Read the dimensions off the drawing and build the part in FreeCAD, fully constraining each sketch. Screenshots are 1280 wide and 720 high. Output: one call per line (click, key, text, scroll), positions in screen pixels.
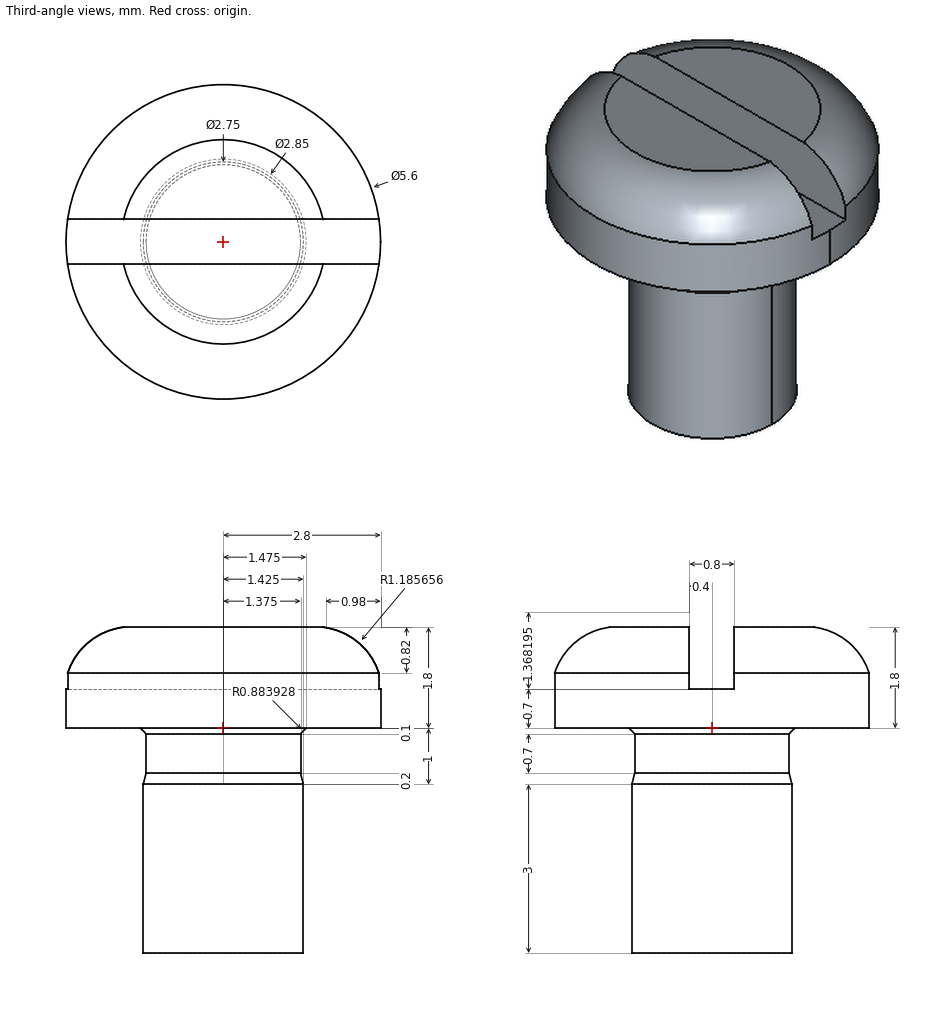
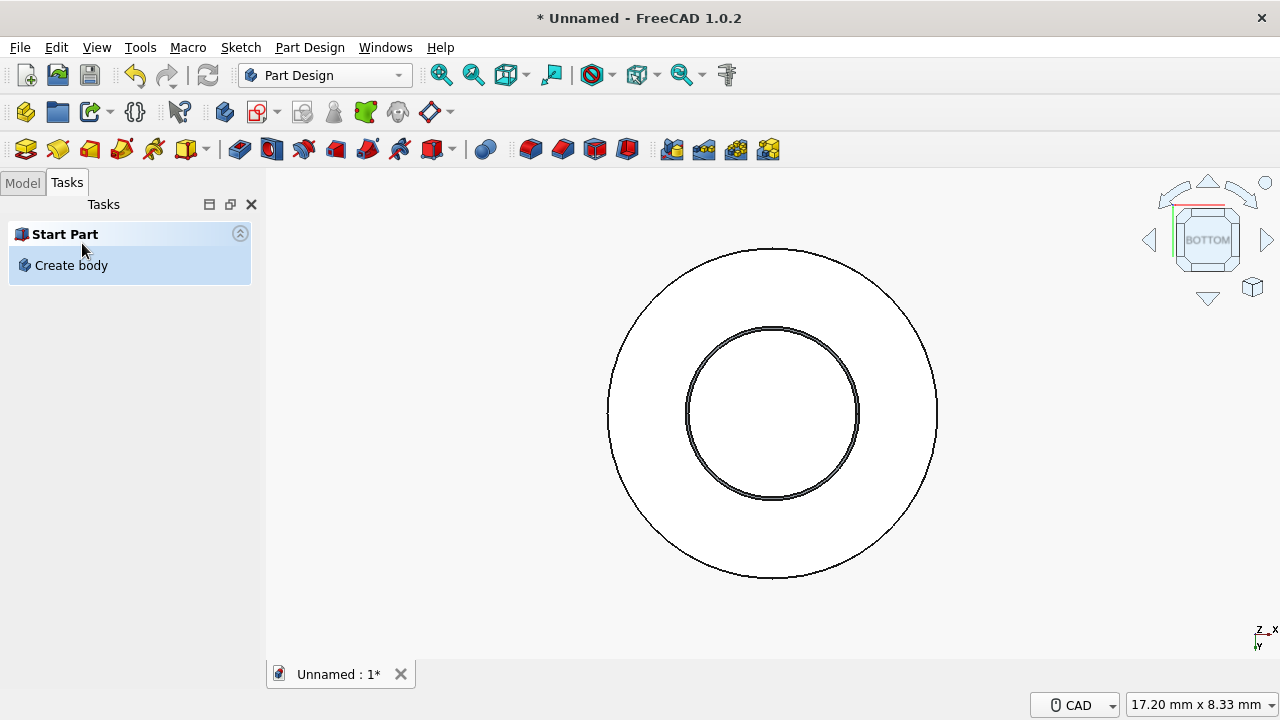
click(23, 182)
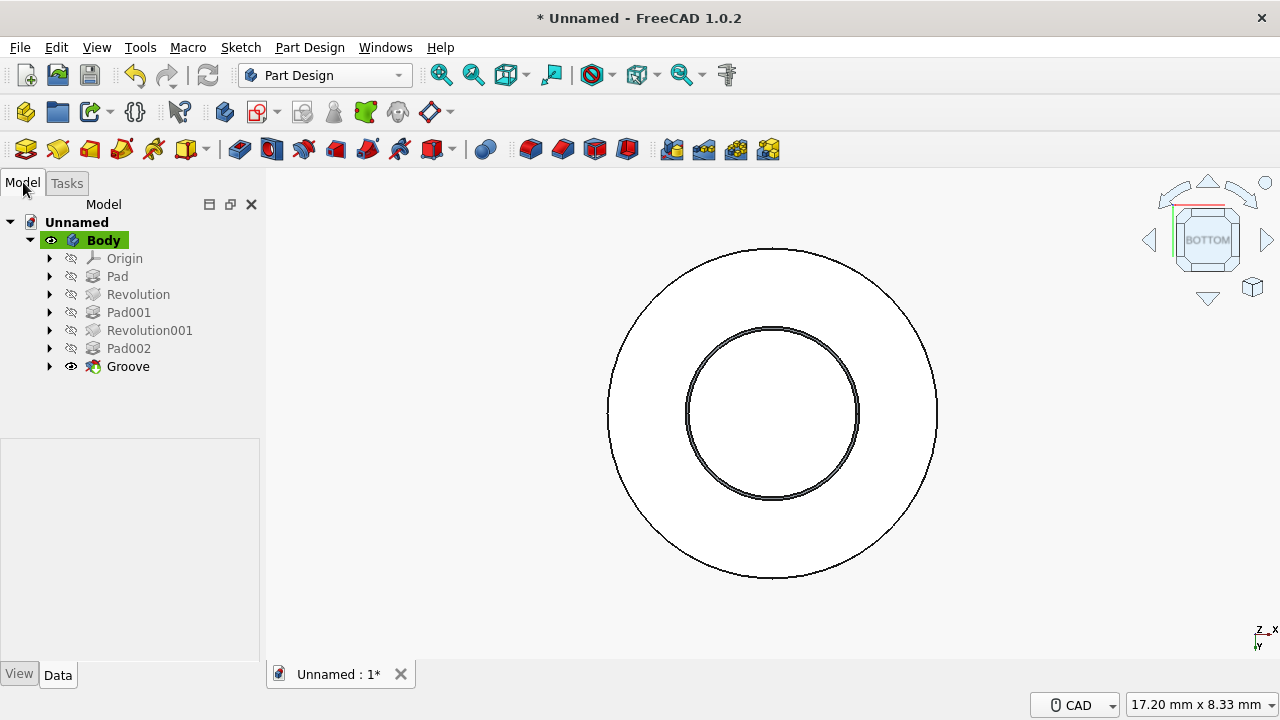
click(50, 258)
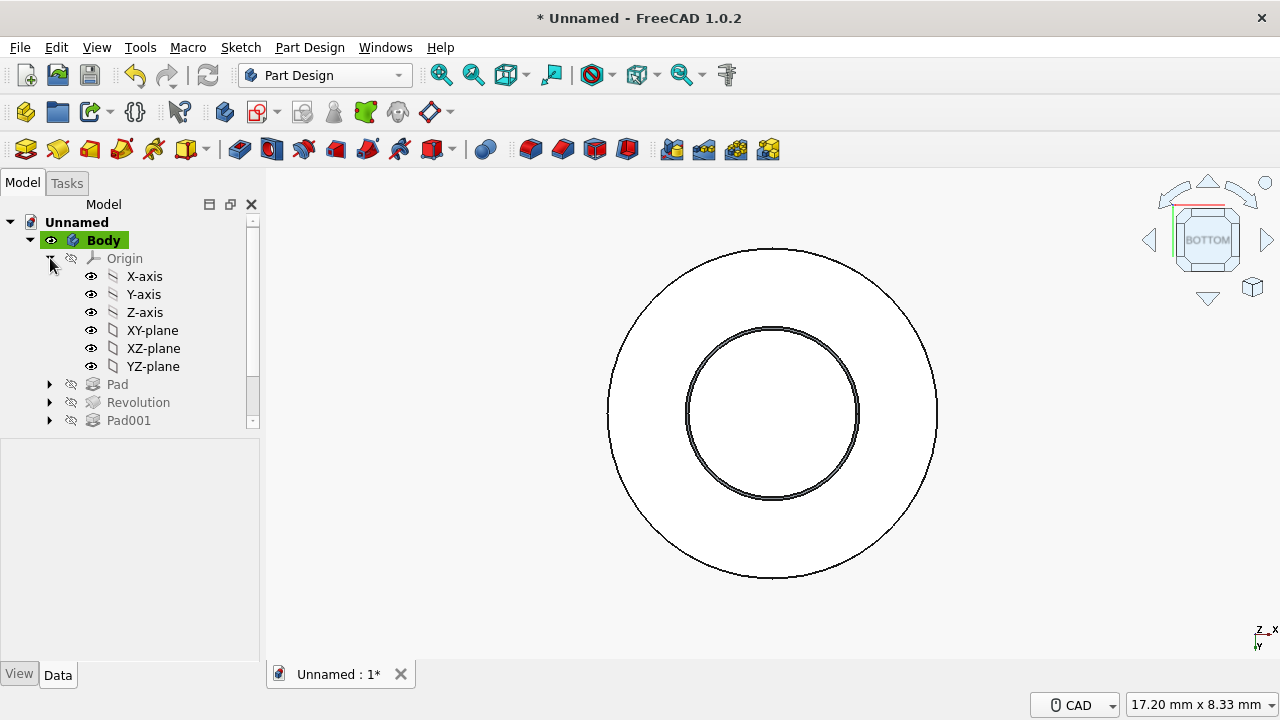
click(136, 366)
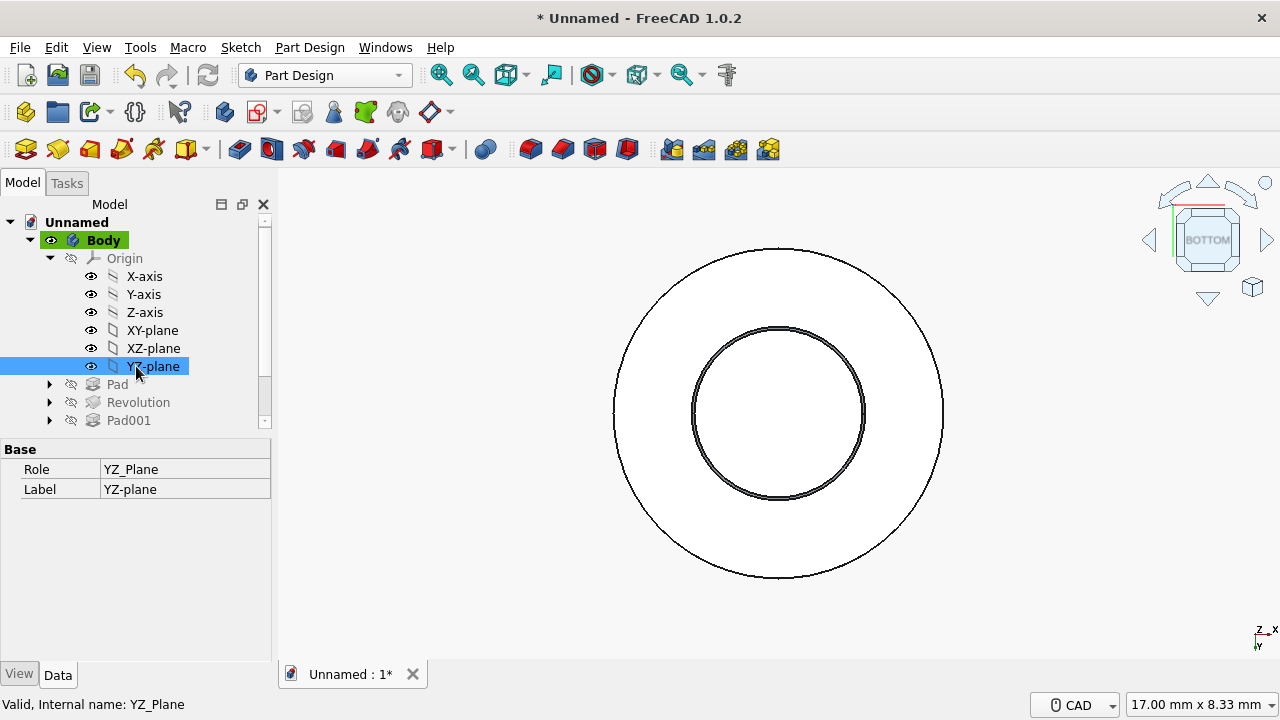
click(430, 112)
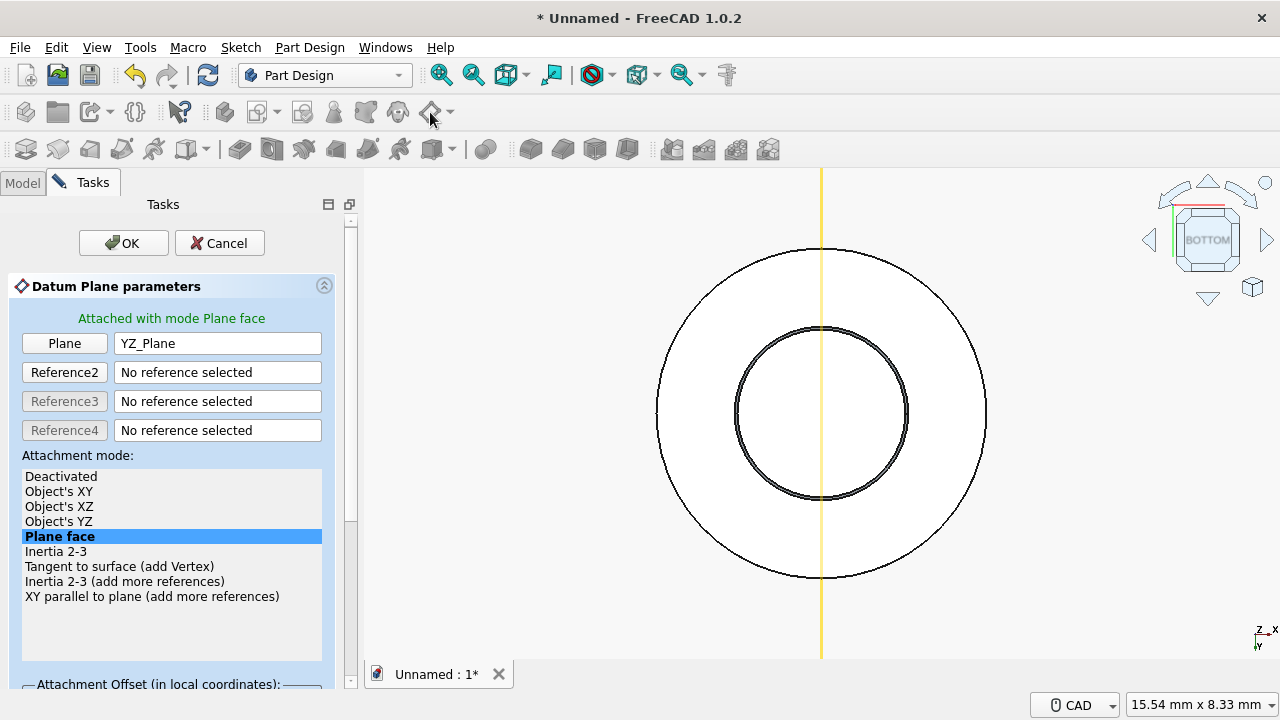
scroll(351, 451, down, 3)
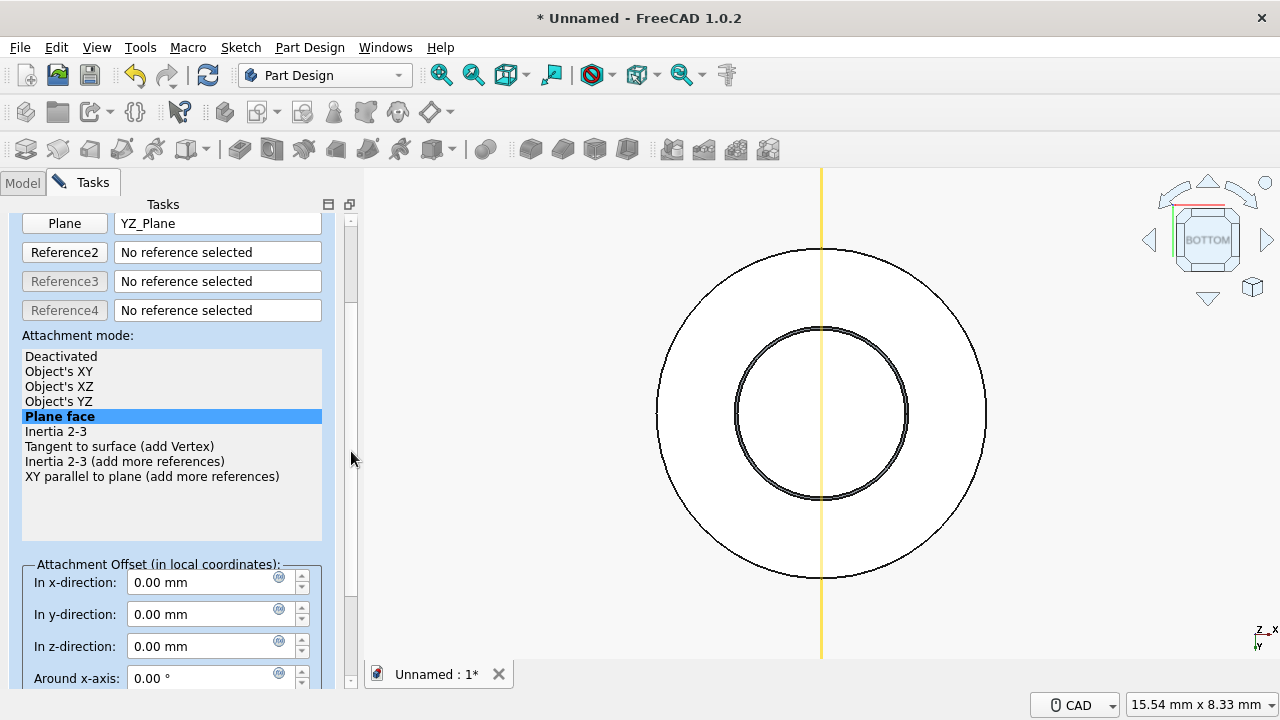
triple_click(210, 586)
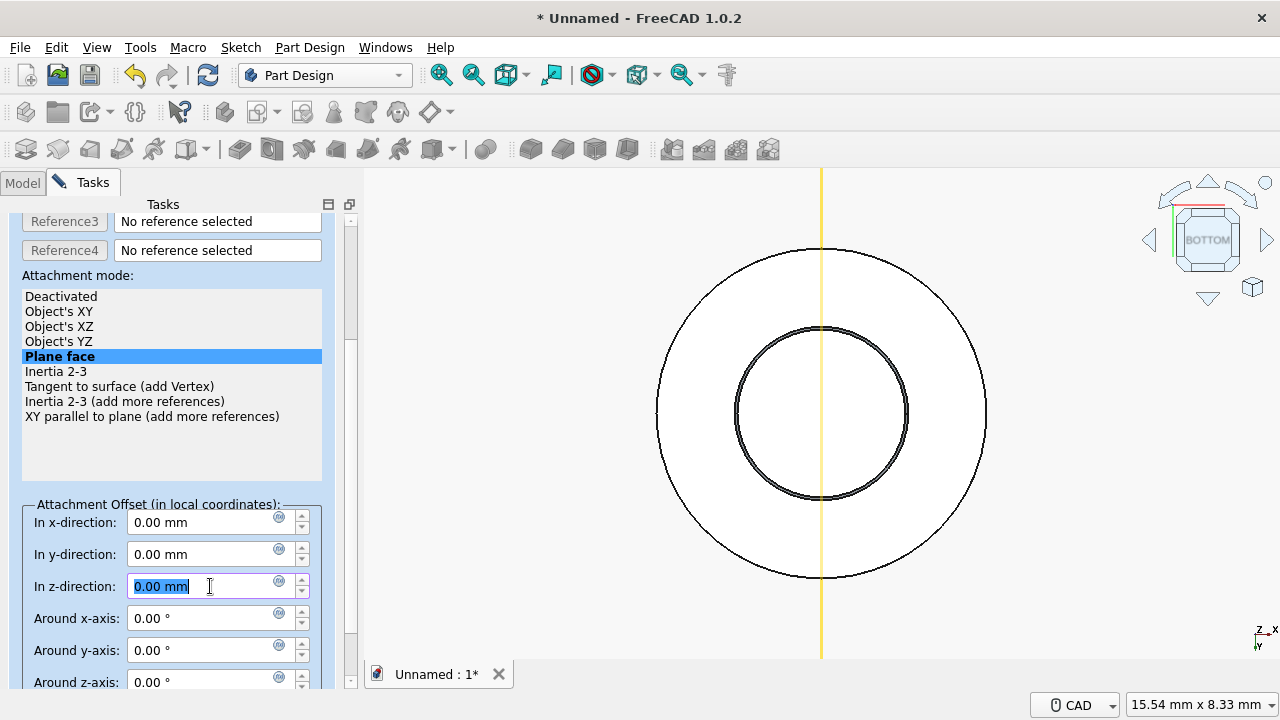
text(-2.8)
key(Tab)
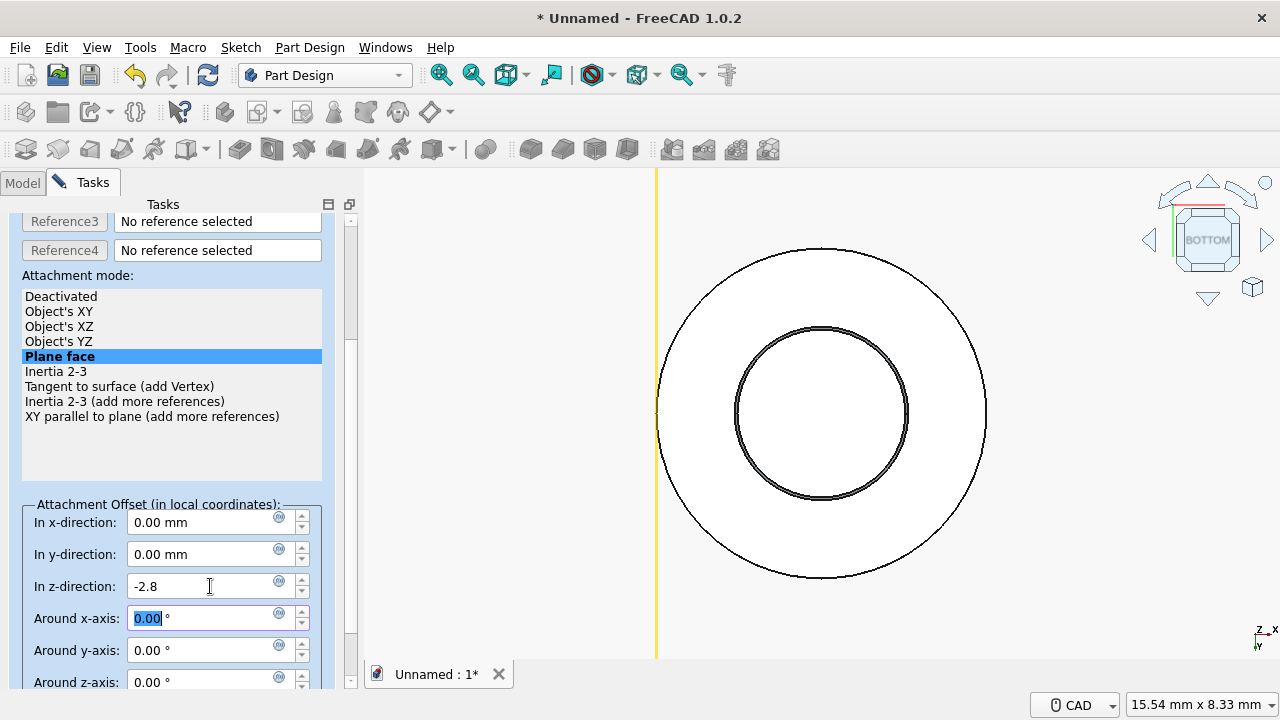
scroll(351, 451, up, 4)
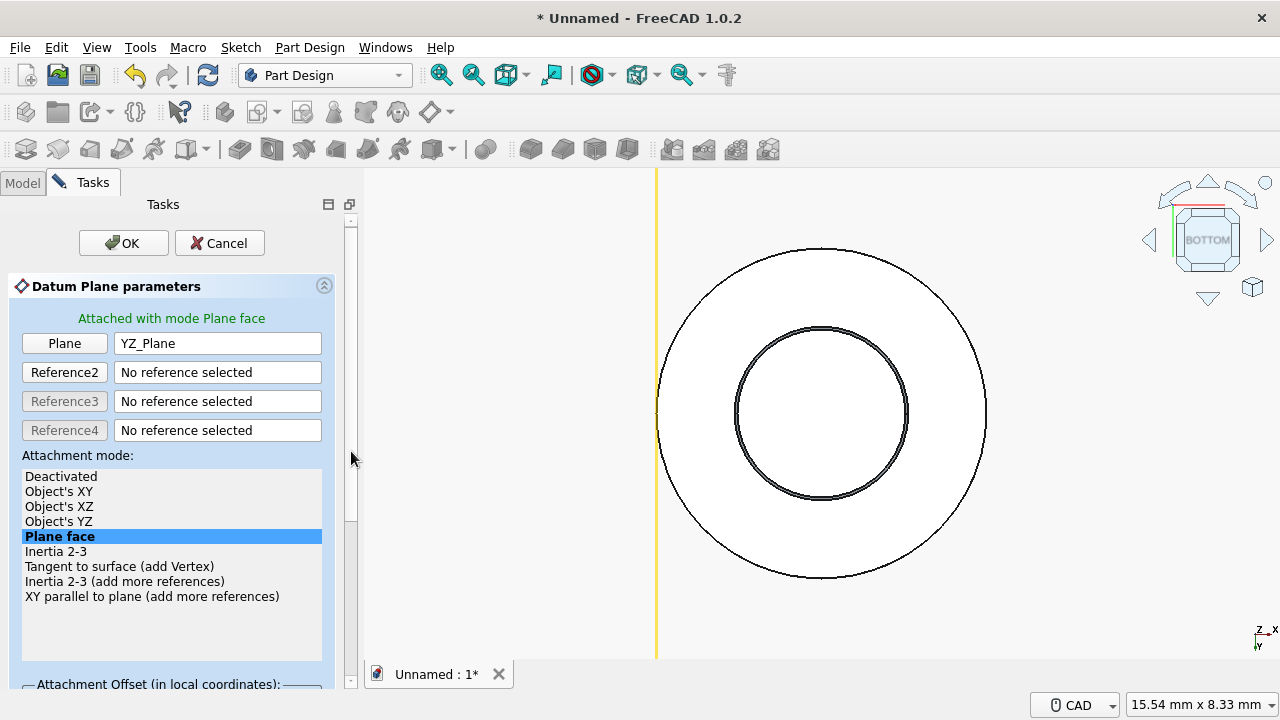
click(124, 243)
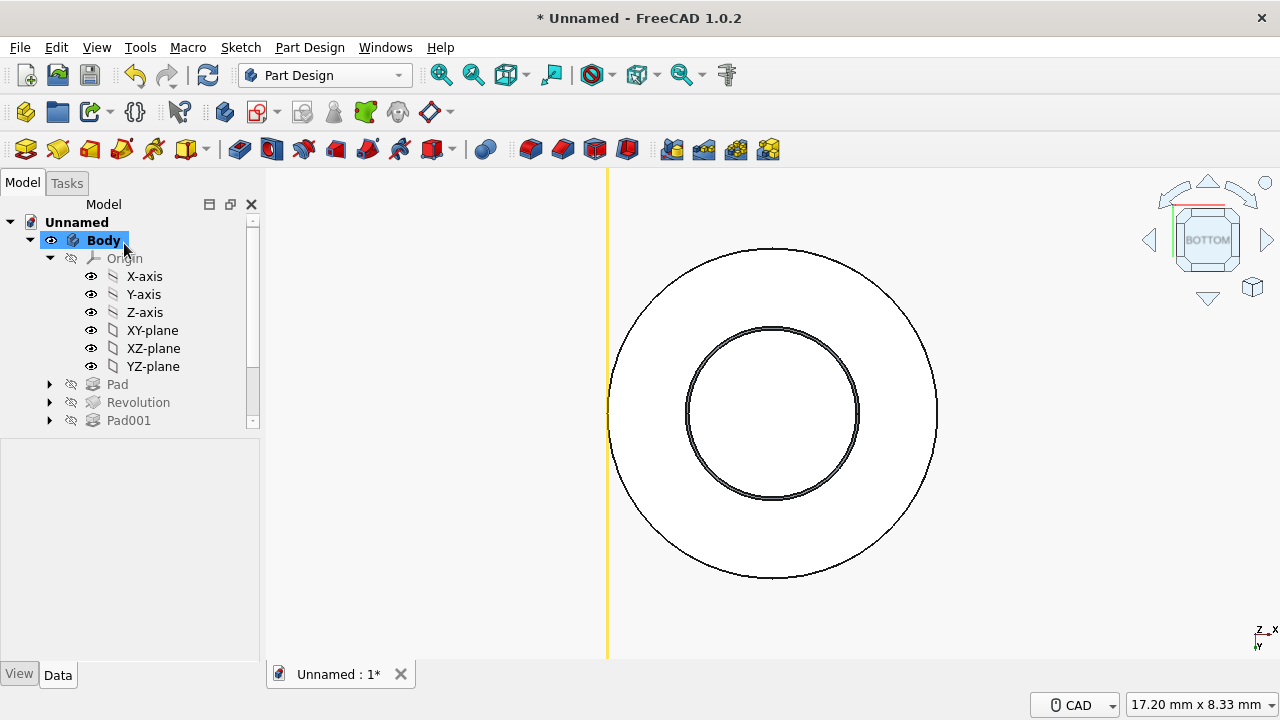
scroll(100, 326, down, 3)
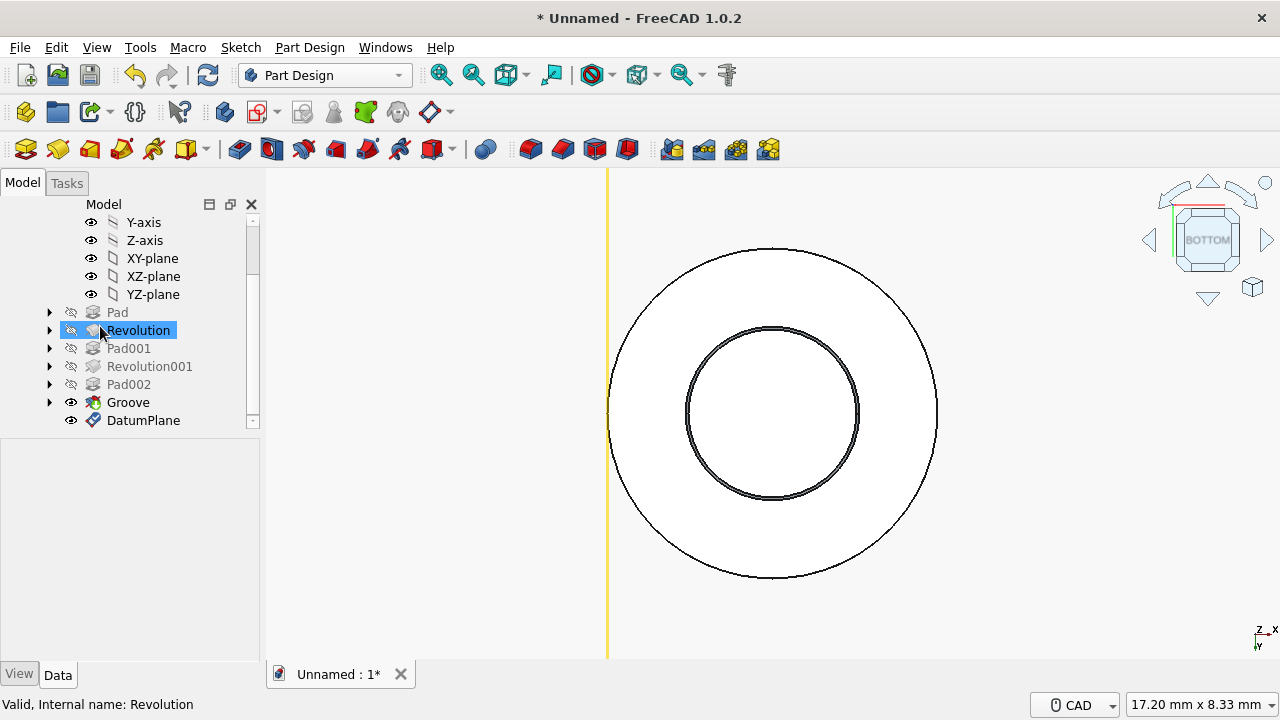
click(116, 420)